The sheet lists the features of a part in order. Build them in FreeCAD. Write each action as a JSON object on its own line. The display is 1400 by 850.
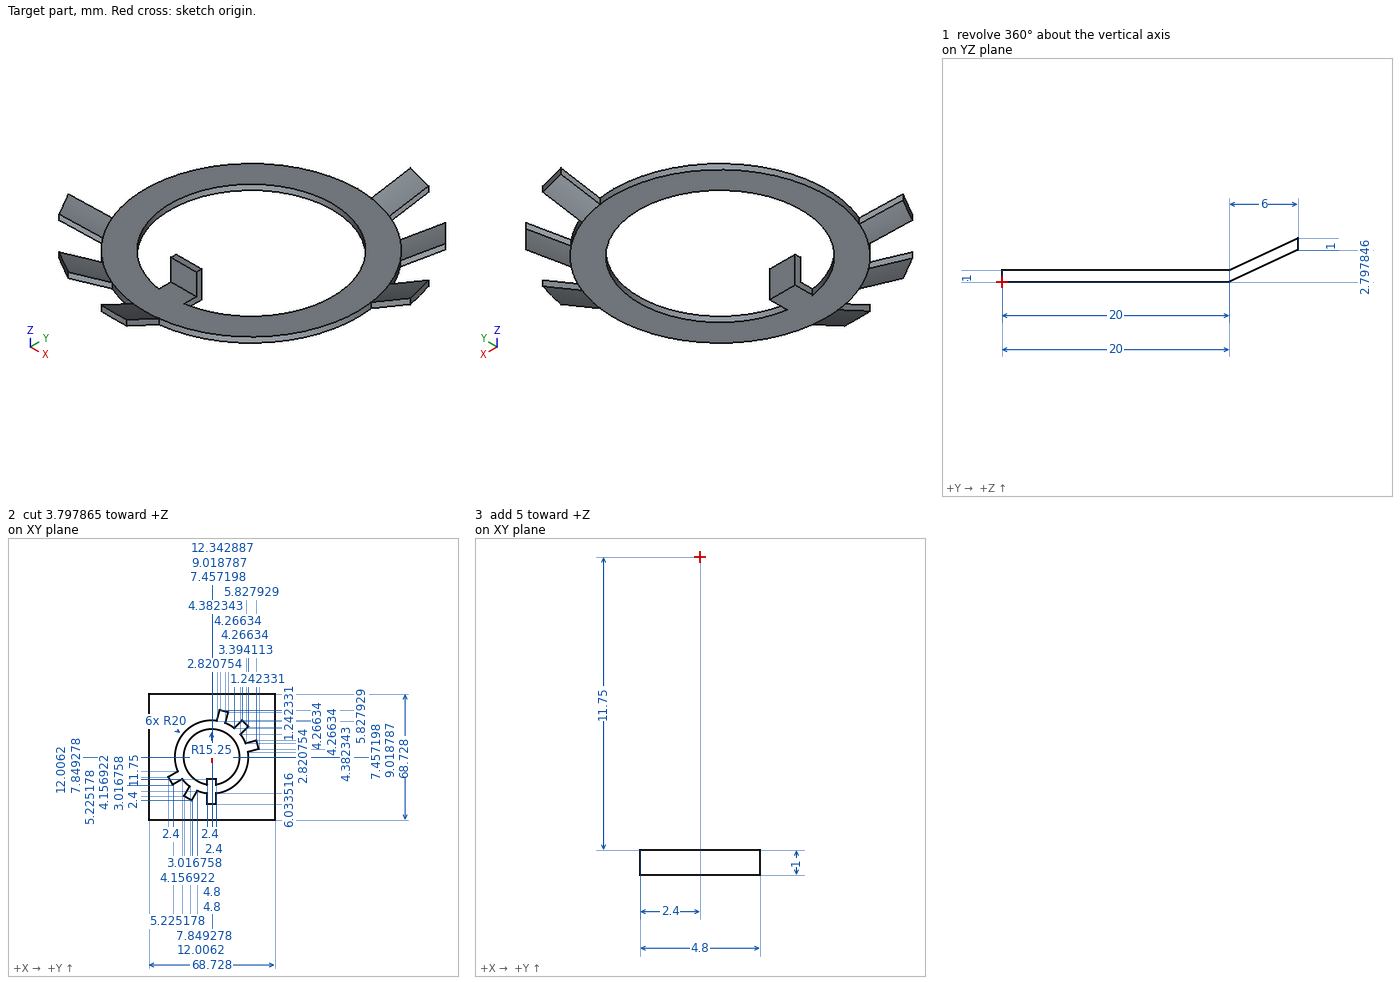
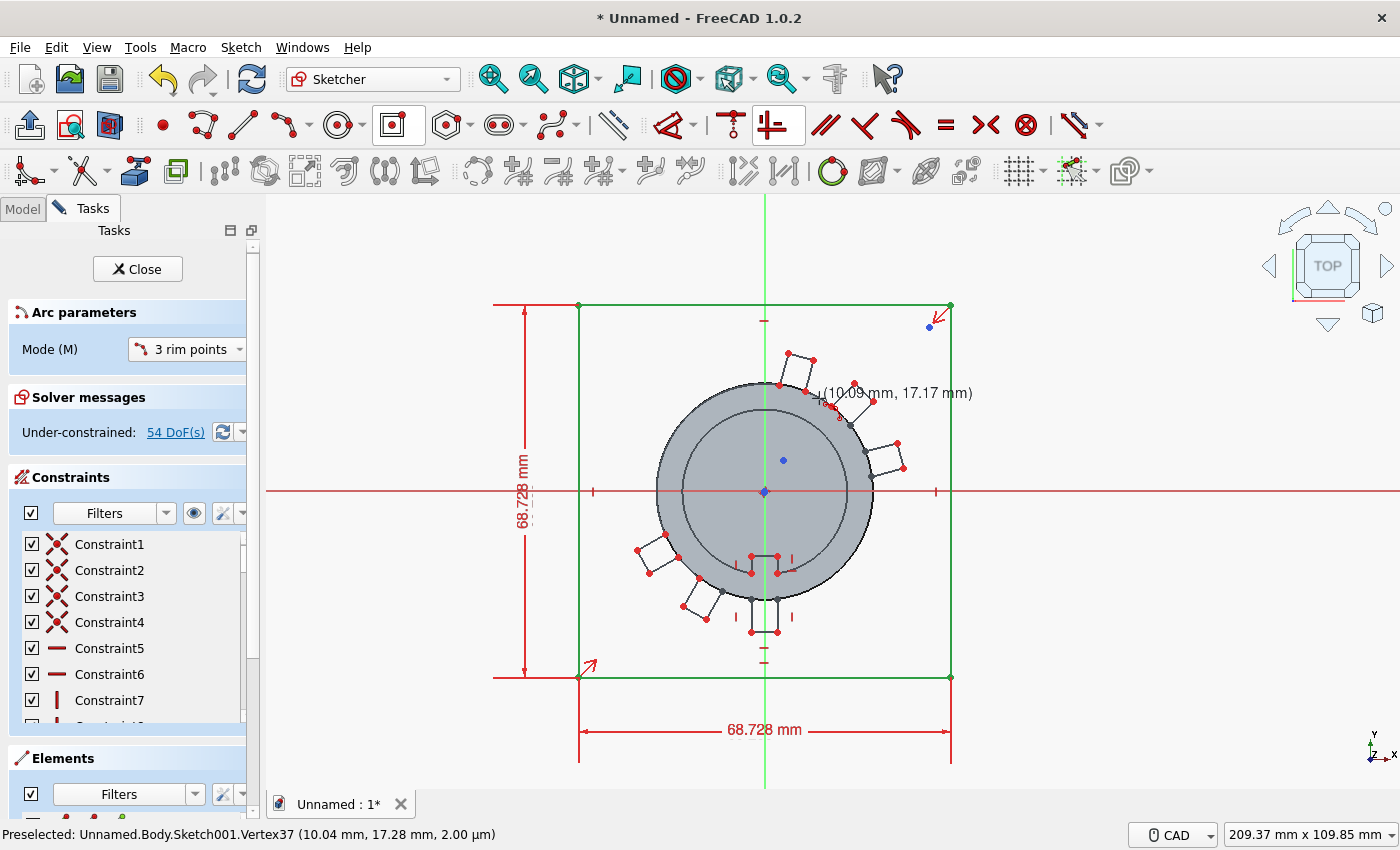
{"action": "left_click", "coordinate": [850, 425]}
{"action": "left_click", "coordinate": [865, 451]}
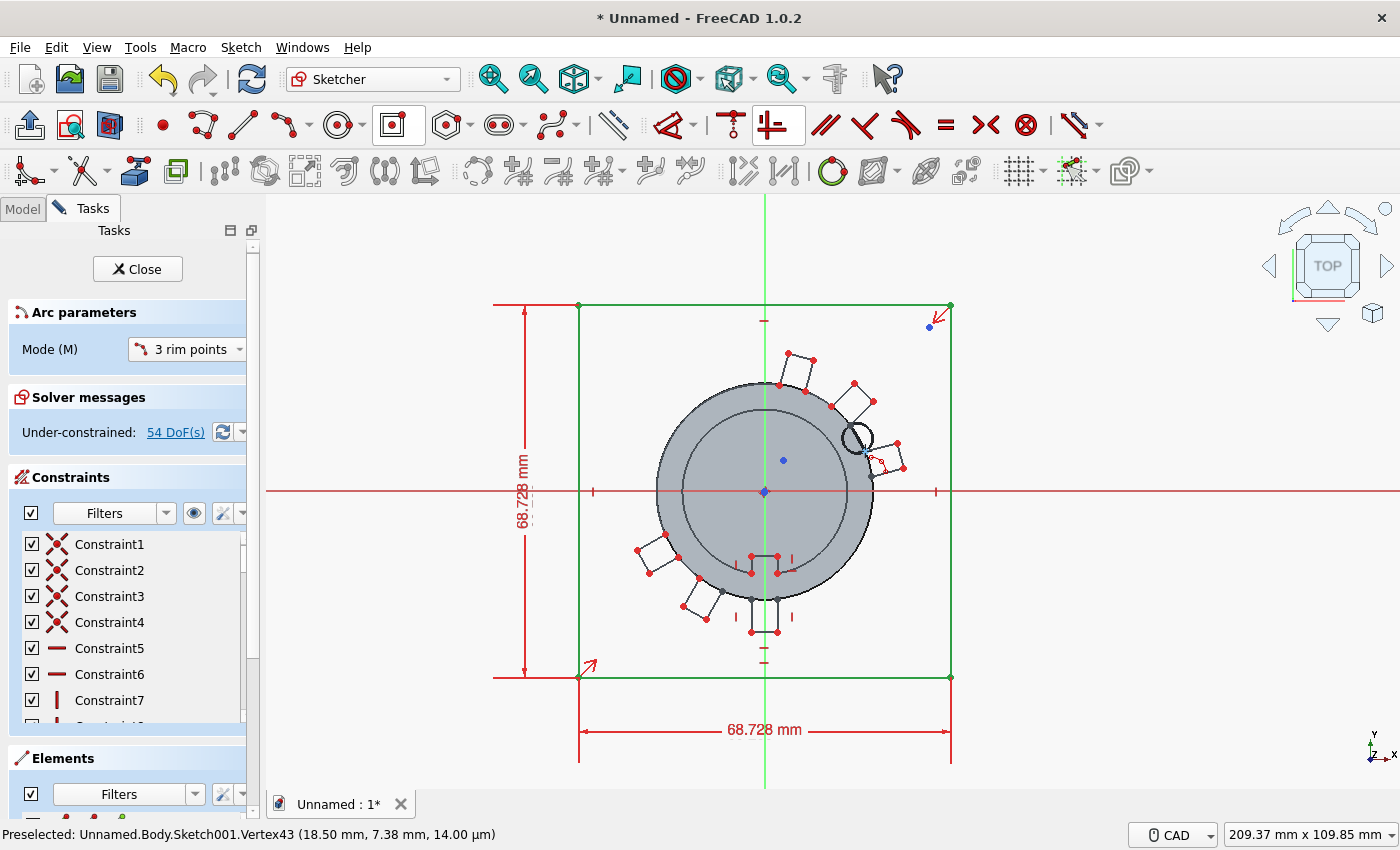
{"action": "scroll", "coordinate": [859, 437], "scroll_direction": "up", "scroll_amount": 14}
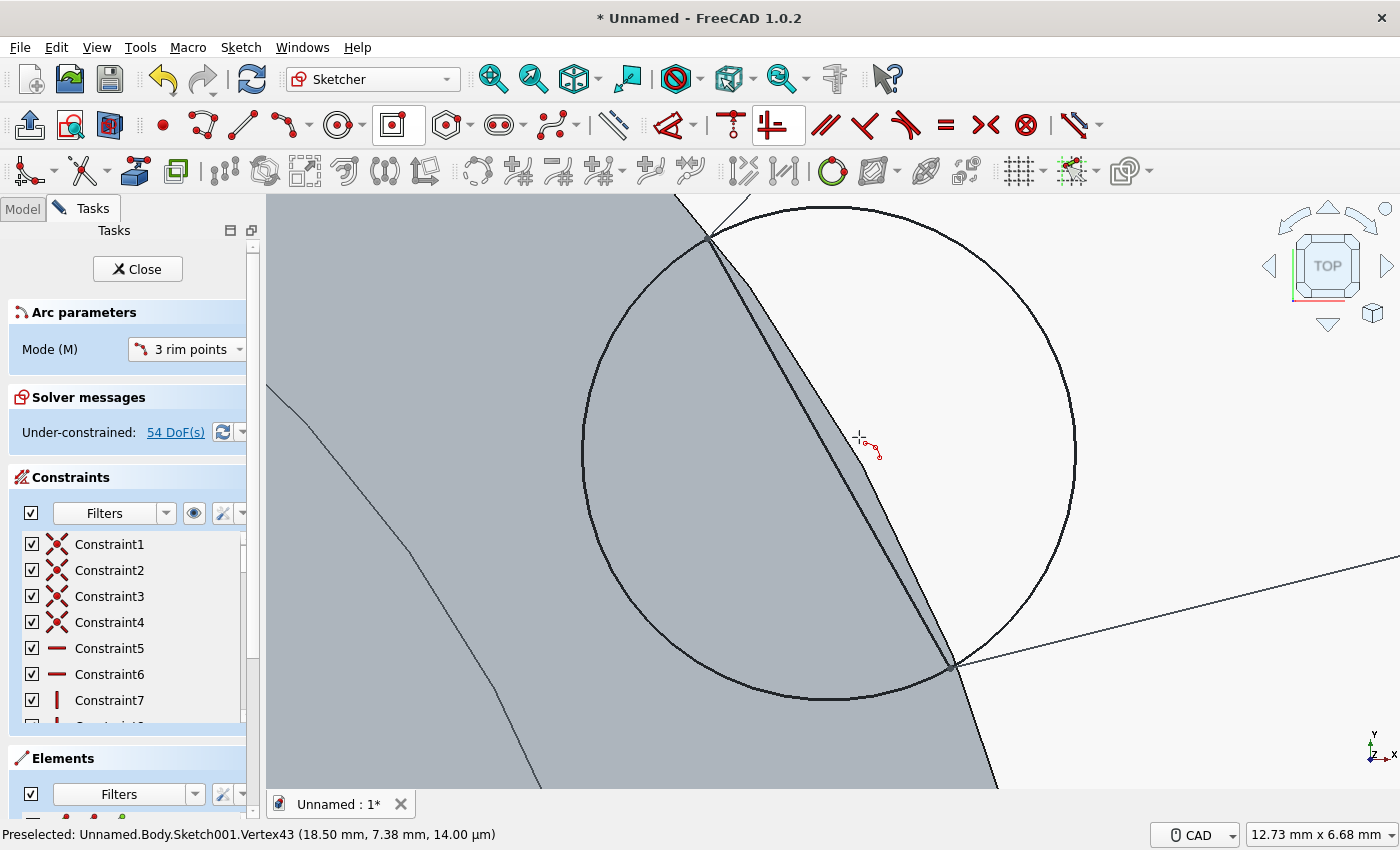
{"action": "left_click", "coordinate": [845, 435]}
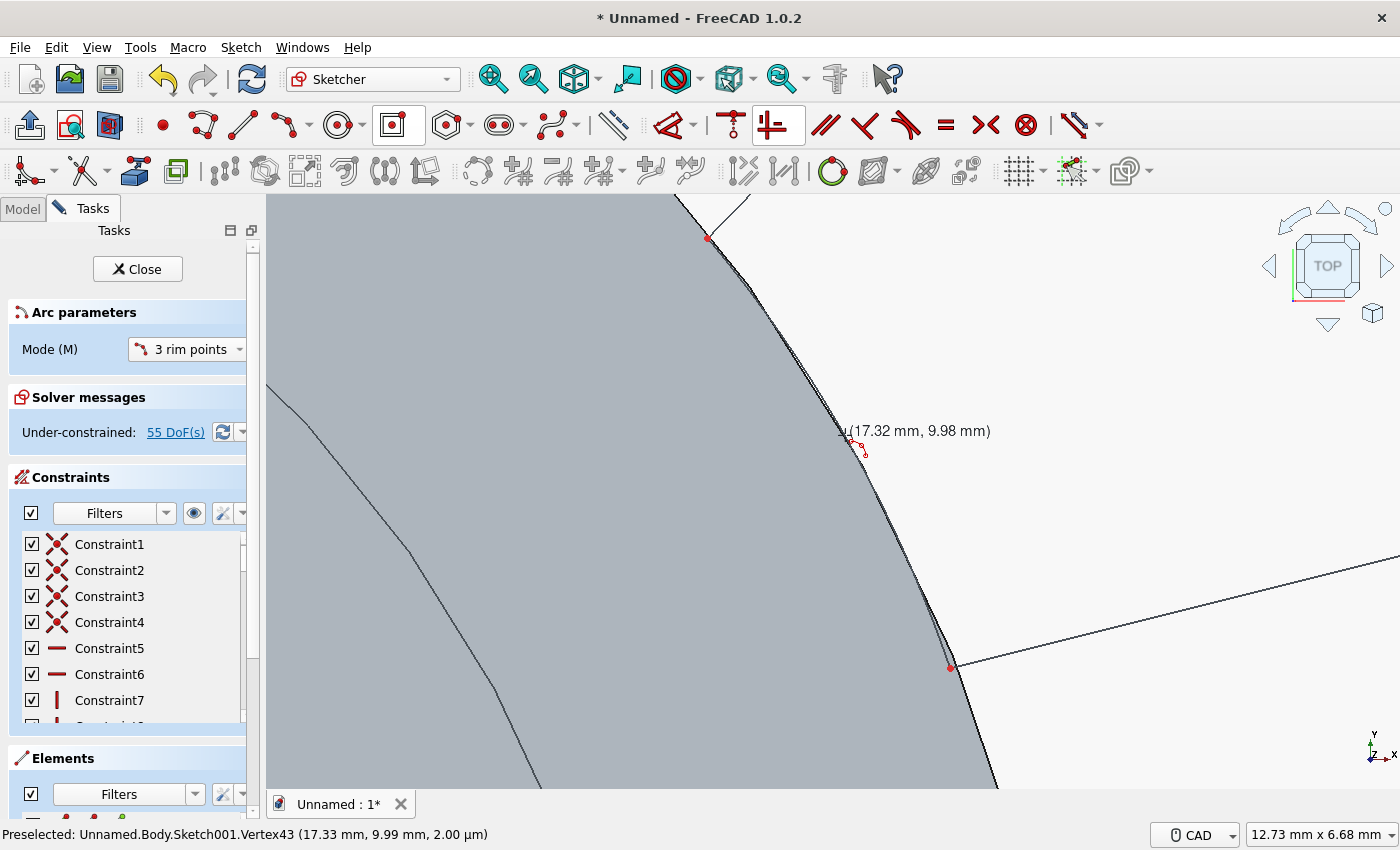
{"action": "scroll", "coordinate": [859, 438], "scroll_direction": "down", "scroll_amount": 14}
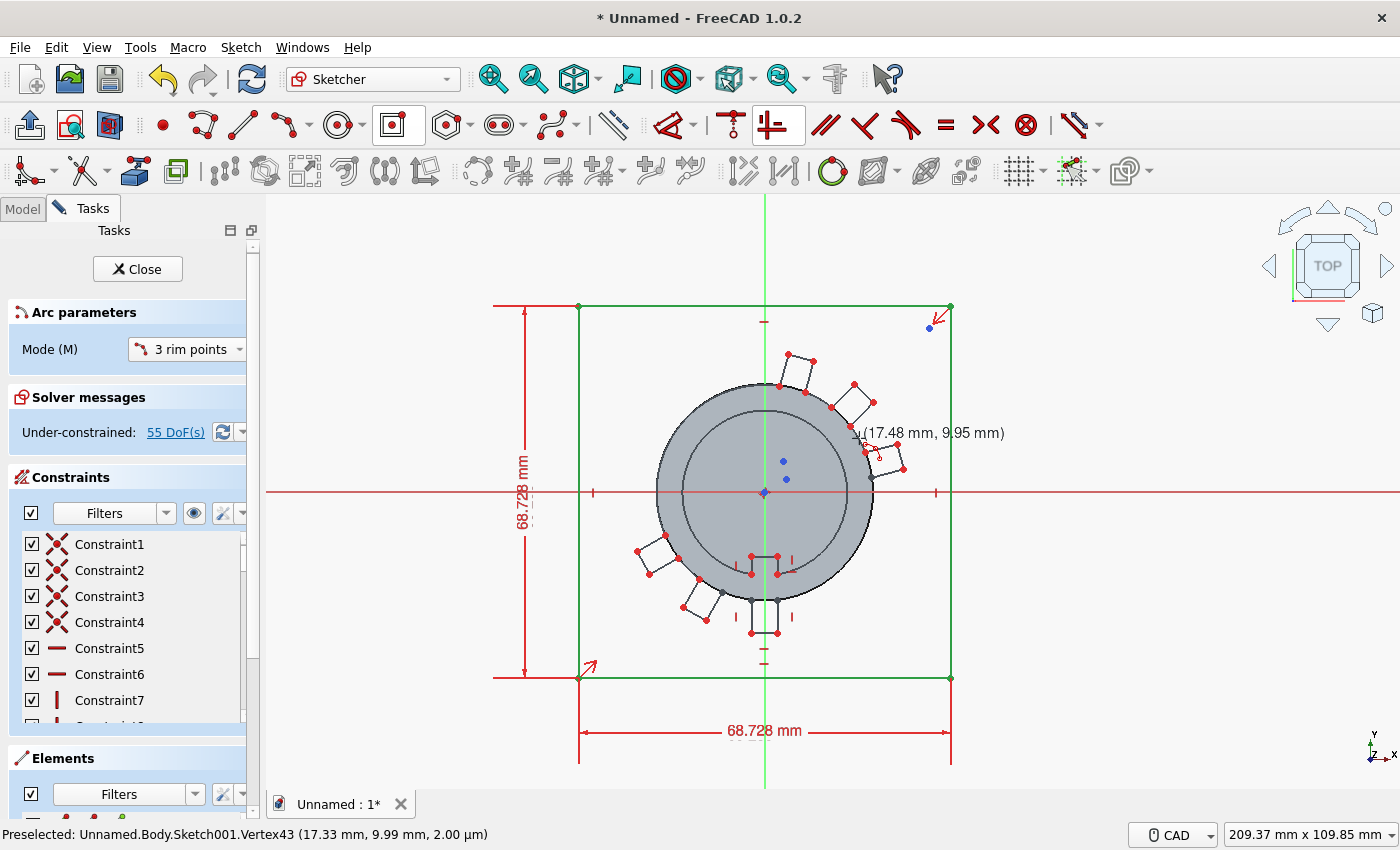
{"action": "left_click", "coordinate": [872, 478]}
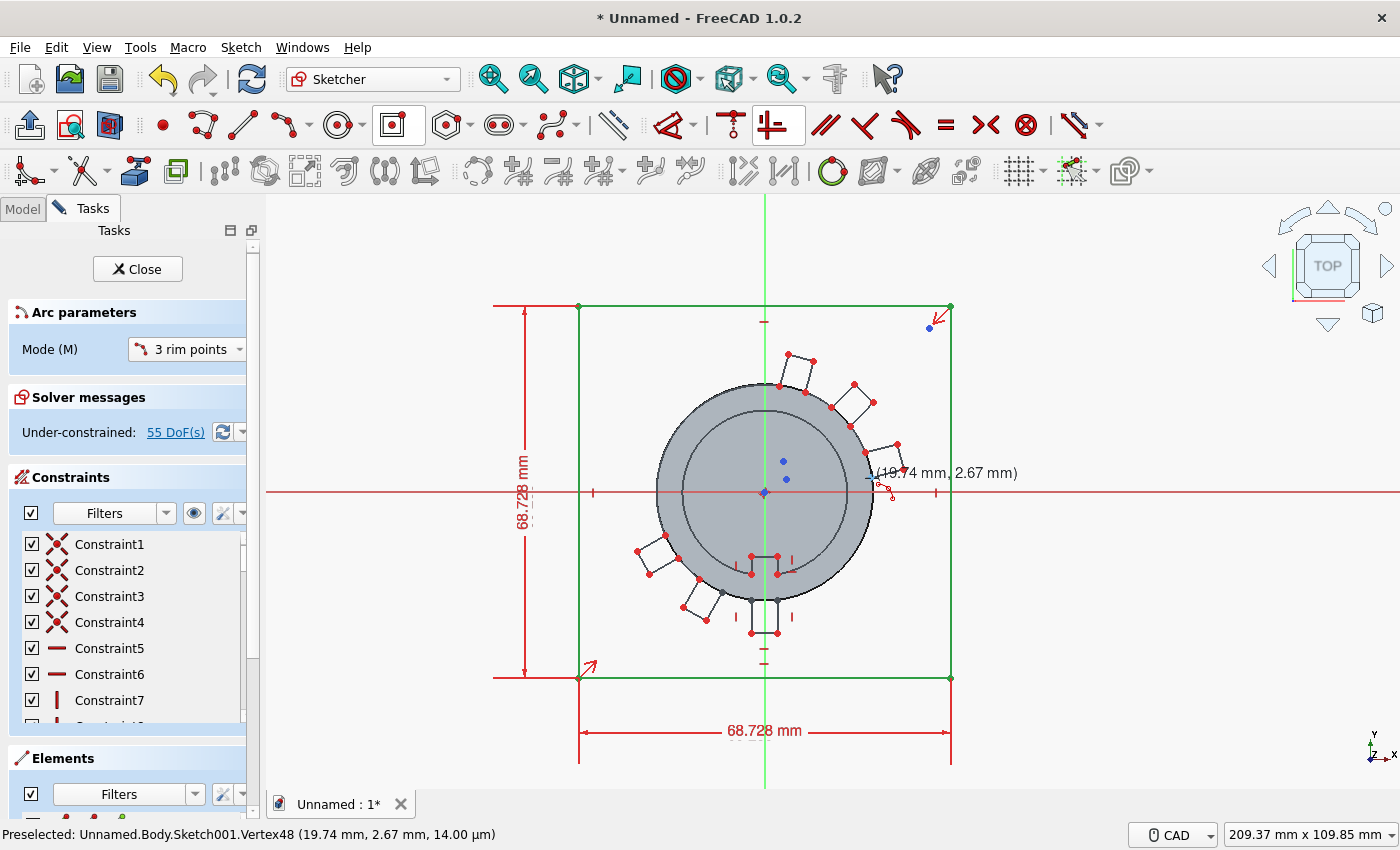
{"action": "scroll", "coordinate": [778, 600], "scroll_direction": "up", "scroll_amount": 2}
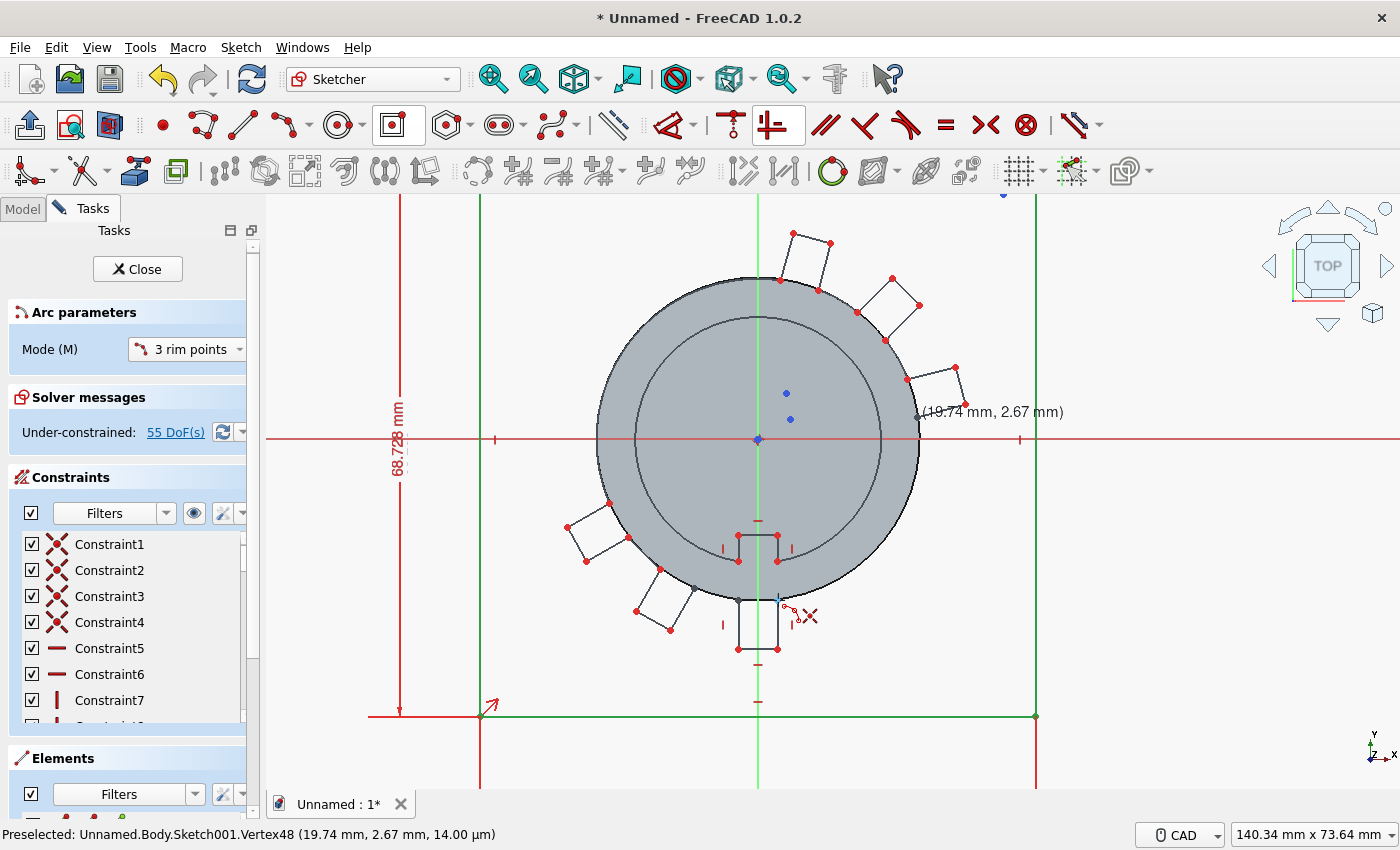
{"action": "left_click", "coordinate": [778, 600]}
{"action": "left_click", "coordinate": [886, 537]}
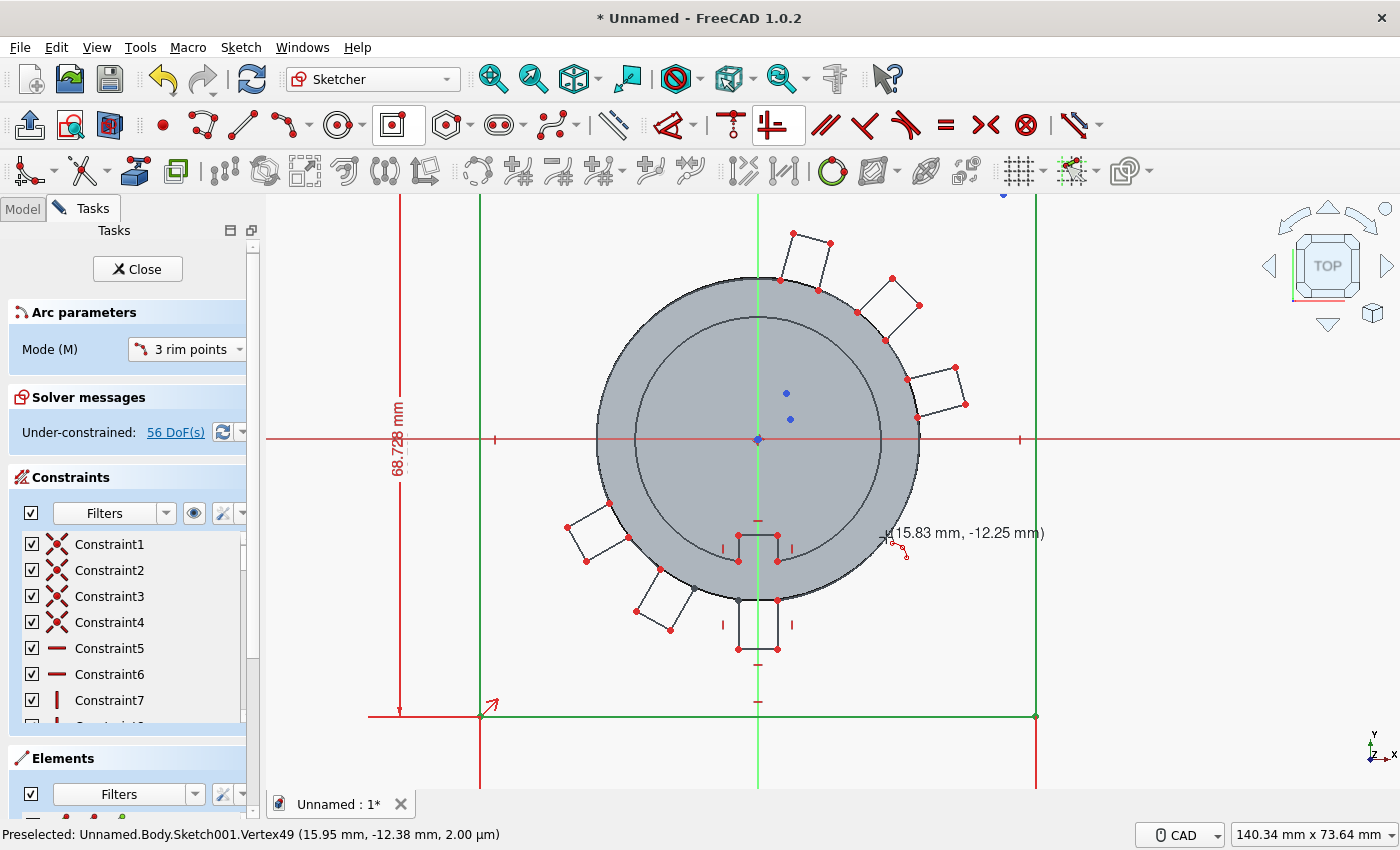
{"action": "left_click", "coordinate": [739, 600]}
{"action": "left_click", "coordinate": [695, 588]}